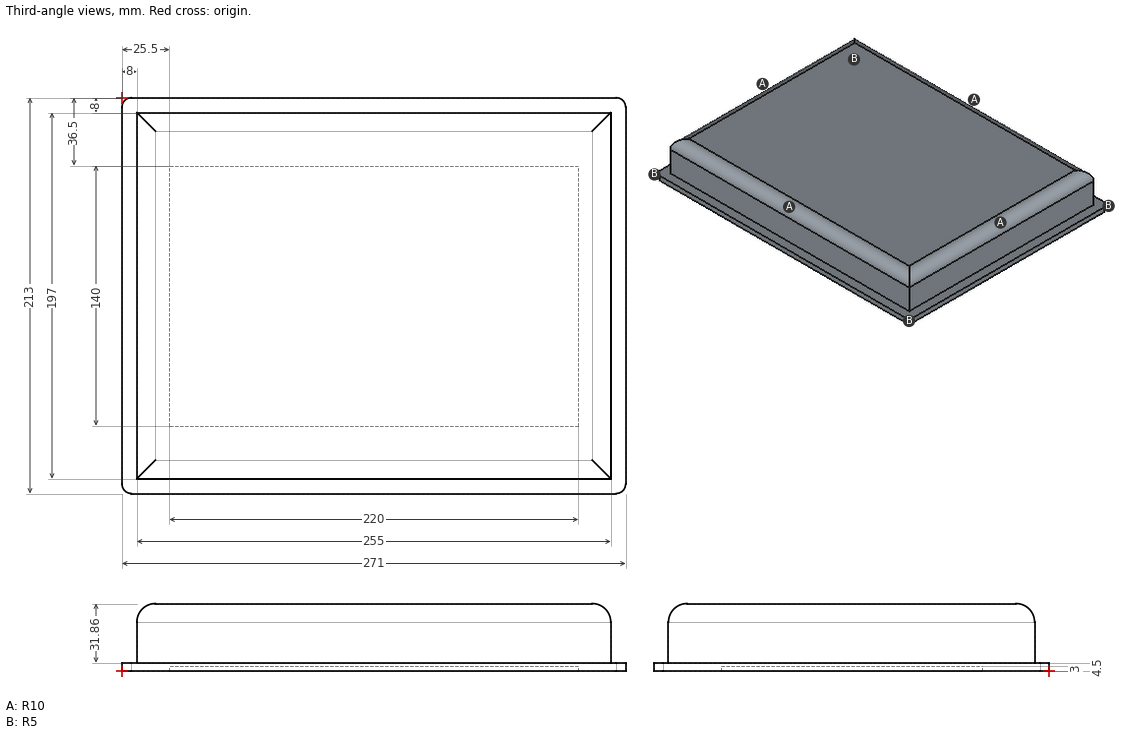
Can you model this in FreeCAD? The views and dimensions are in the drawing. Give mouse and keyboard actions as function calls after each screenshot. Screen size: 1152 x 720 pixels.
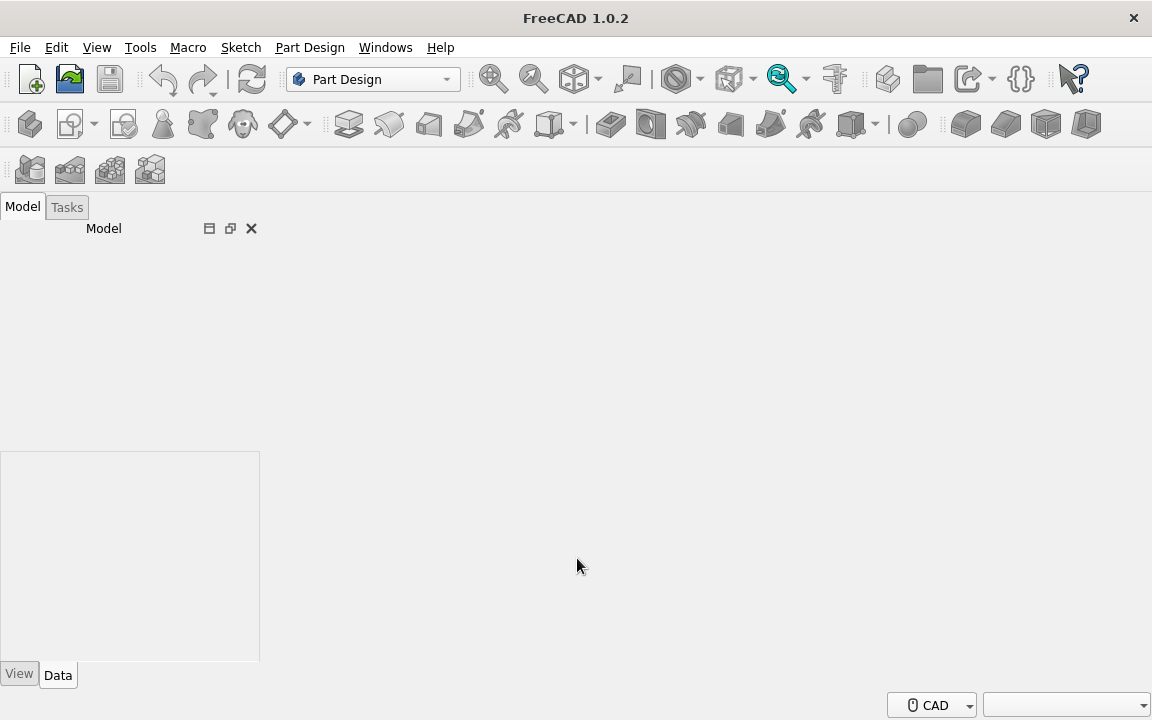
click(30, 80)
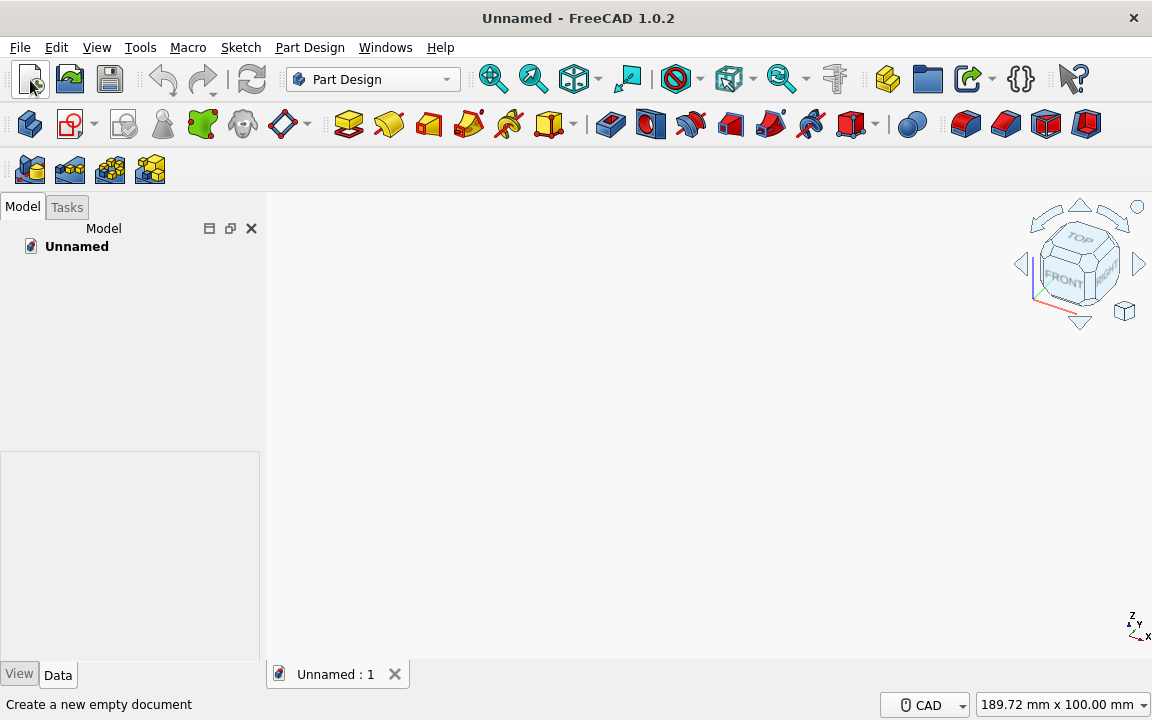
click(70, 124)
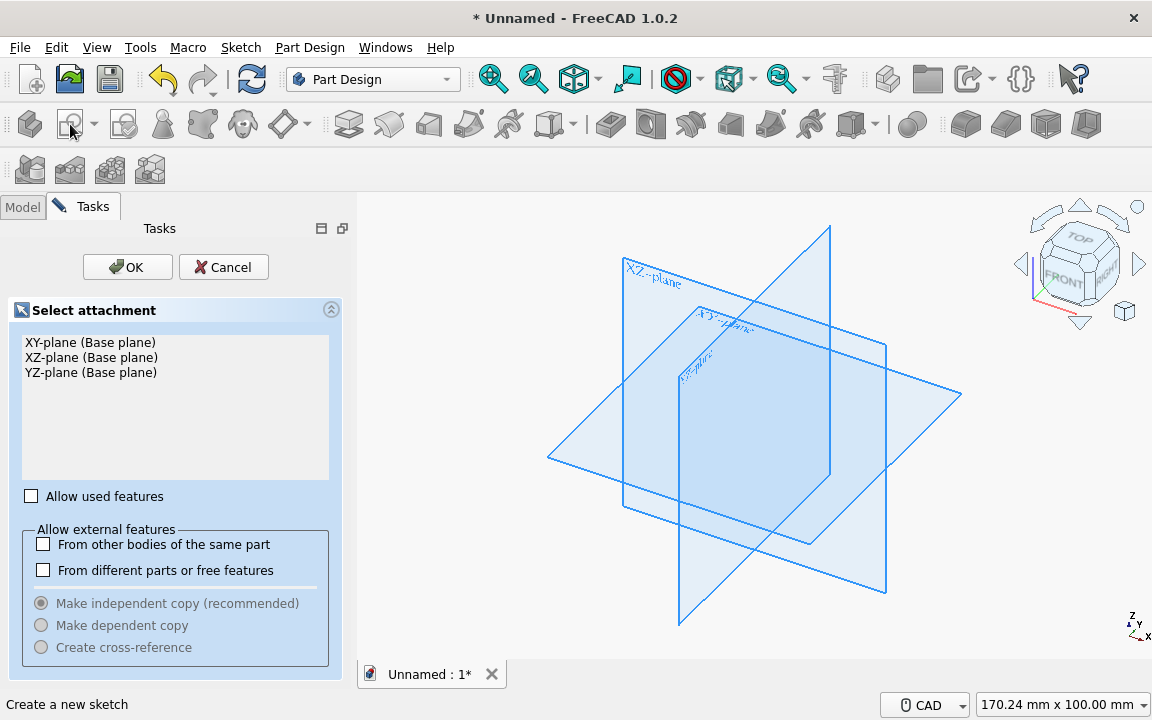
click(82, 342)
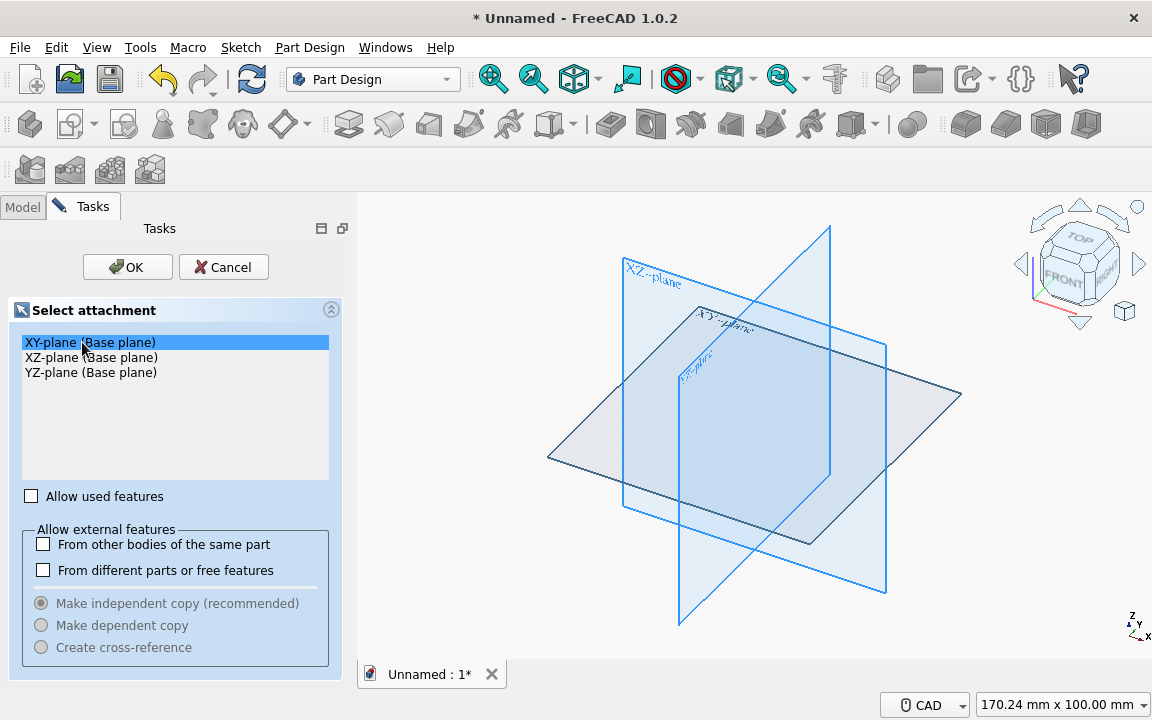
click(128, 267)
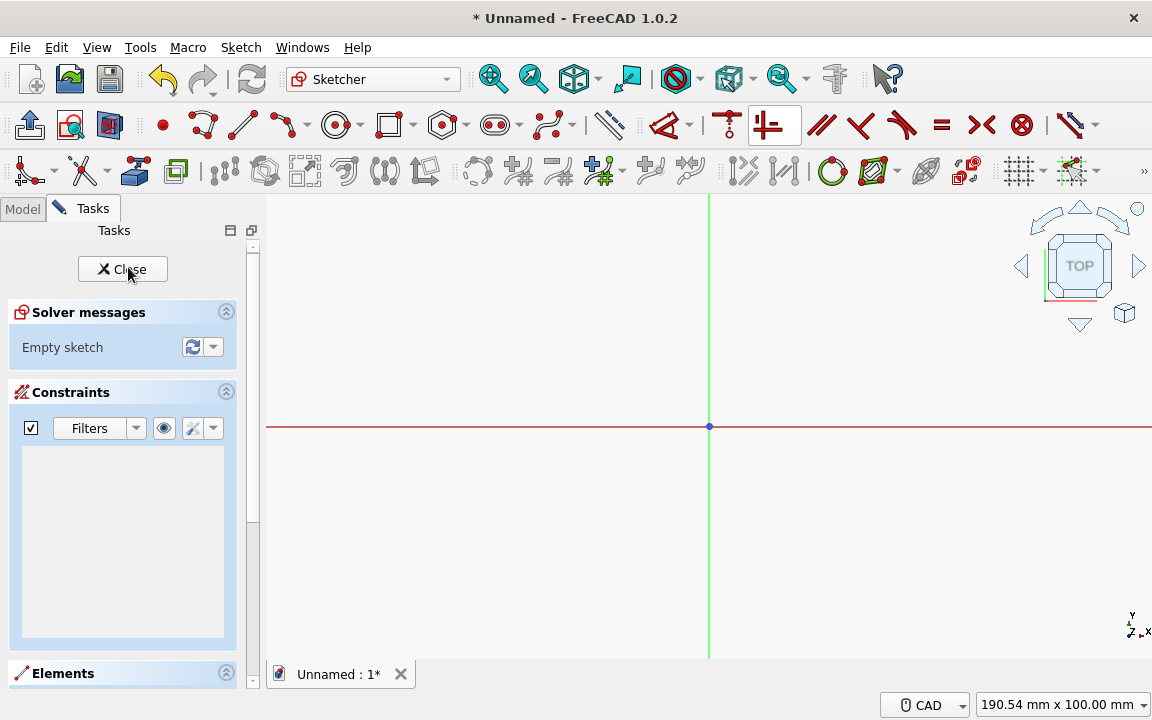
scroll(339, 222, down, 6)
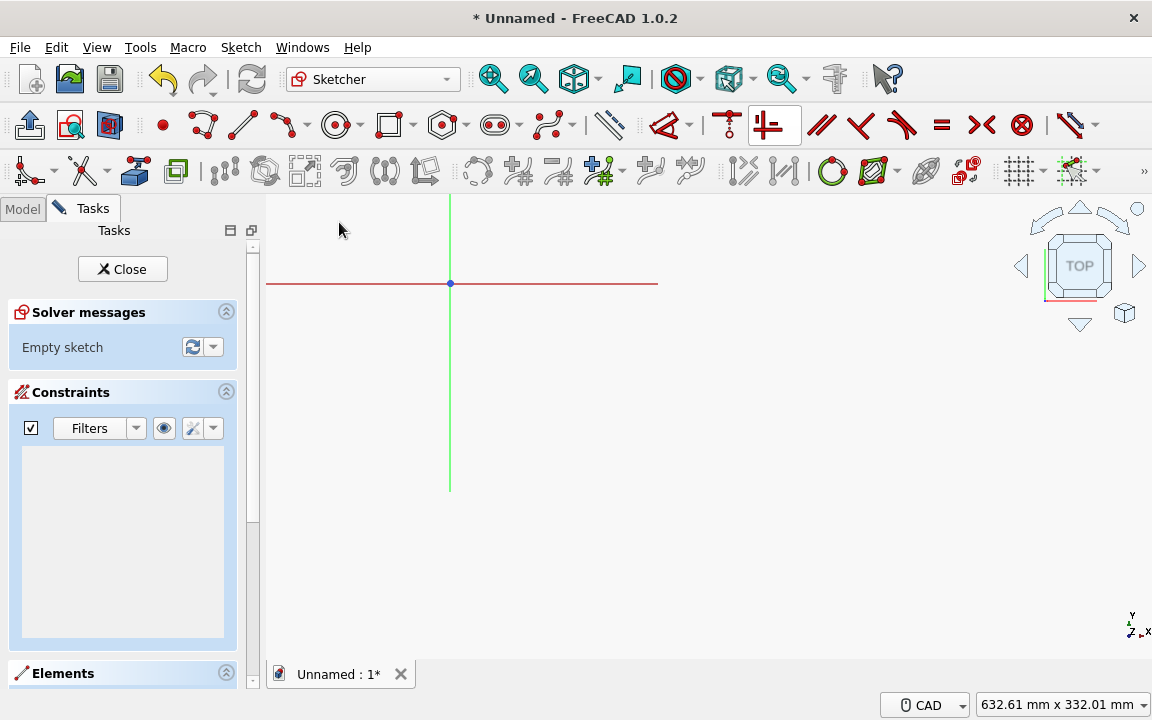
click(390, 126)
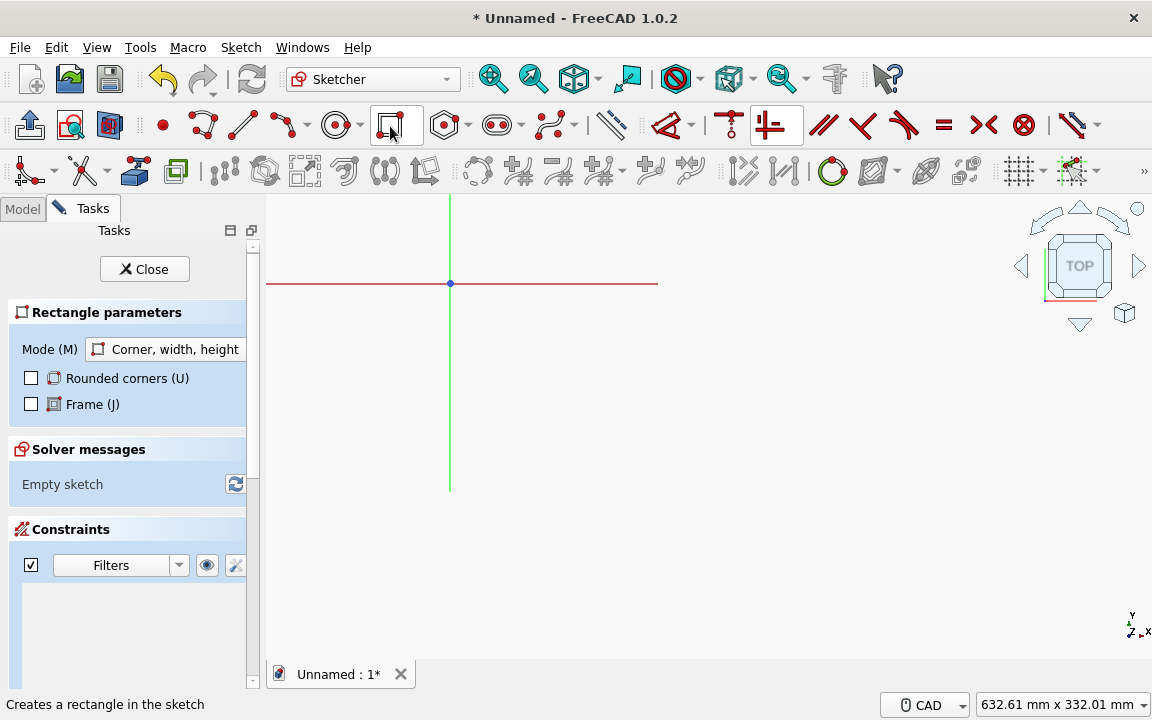
click(450, 284)
click(830, 582)
key(Escape)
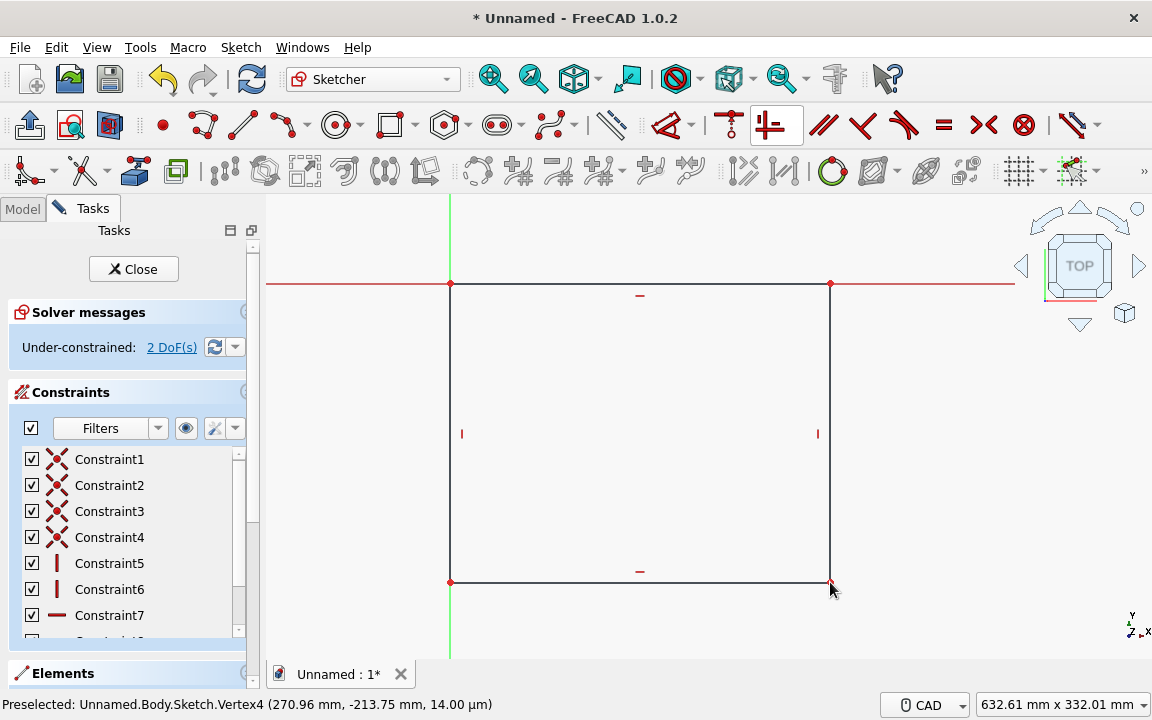
click(666, 126)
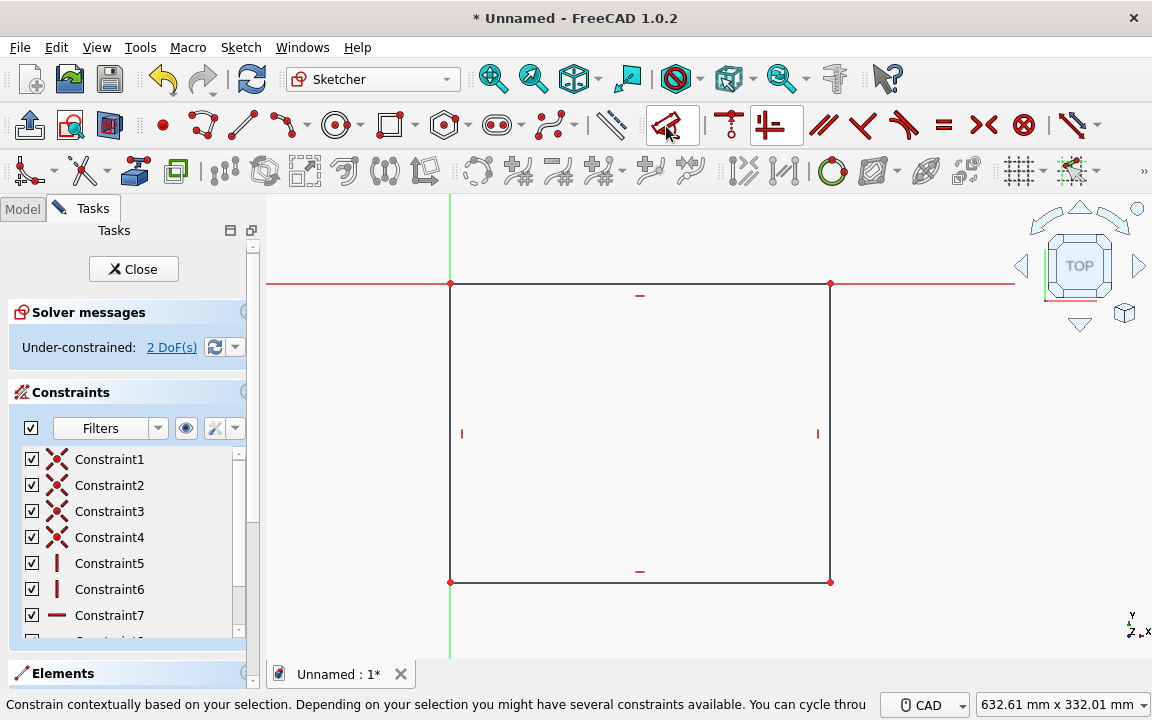
click(450, 373)
click(416, 433)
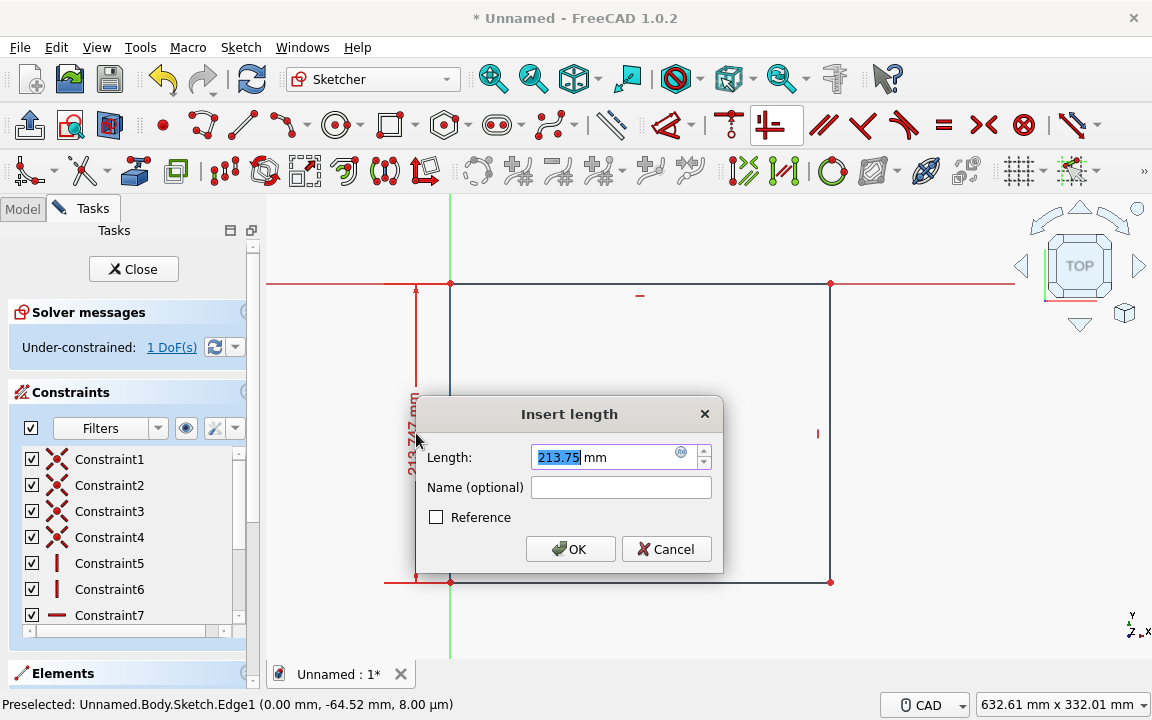
text(213)
key(Return)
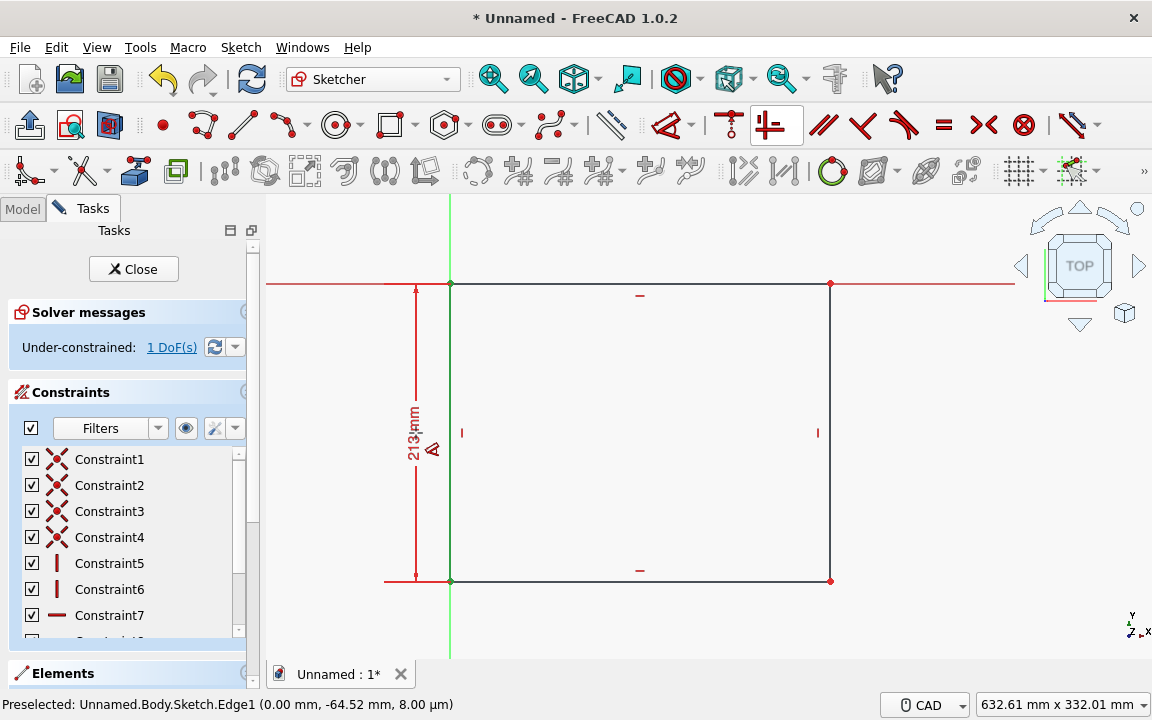
click(564, 582)
click(640, 616)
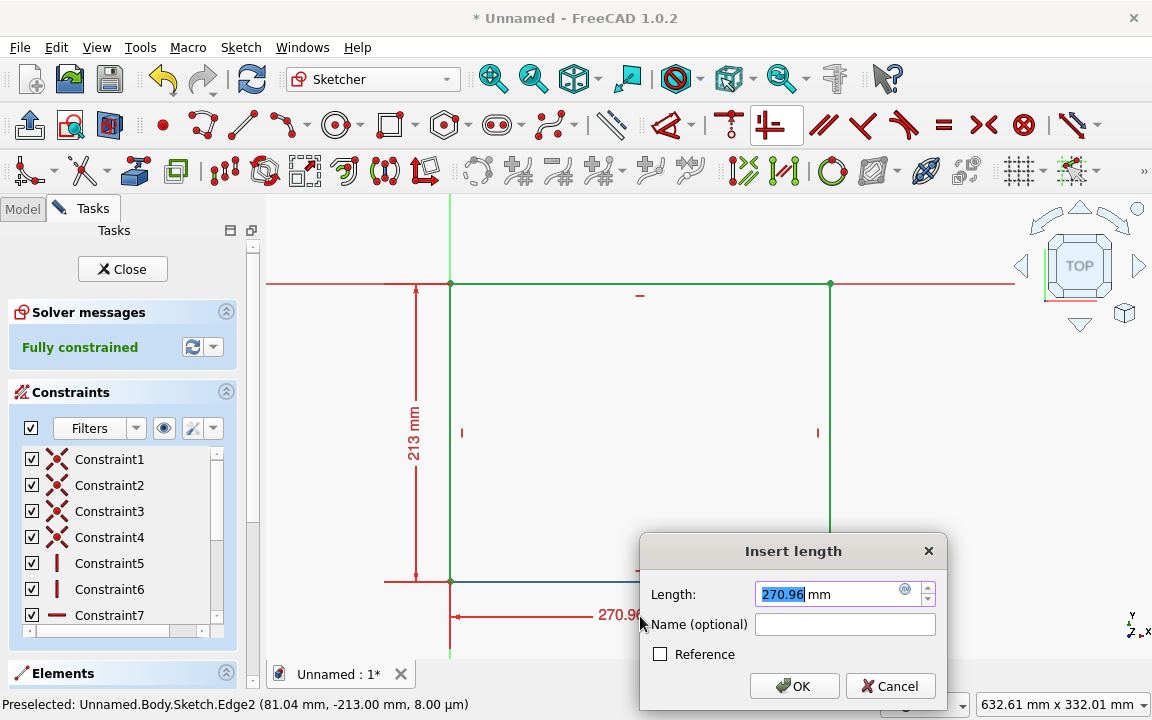
text(271)
key(Return)
key(Escape)